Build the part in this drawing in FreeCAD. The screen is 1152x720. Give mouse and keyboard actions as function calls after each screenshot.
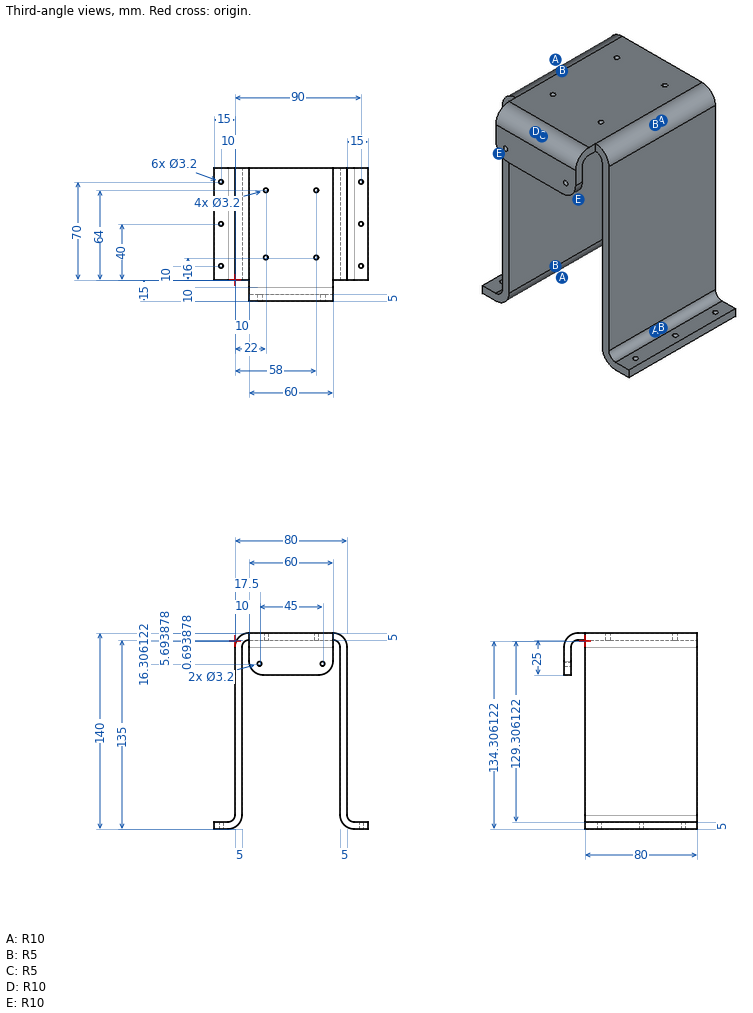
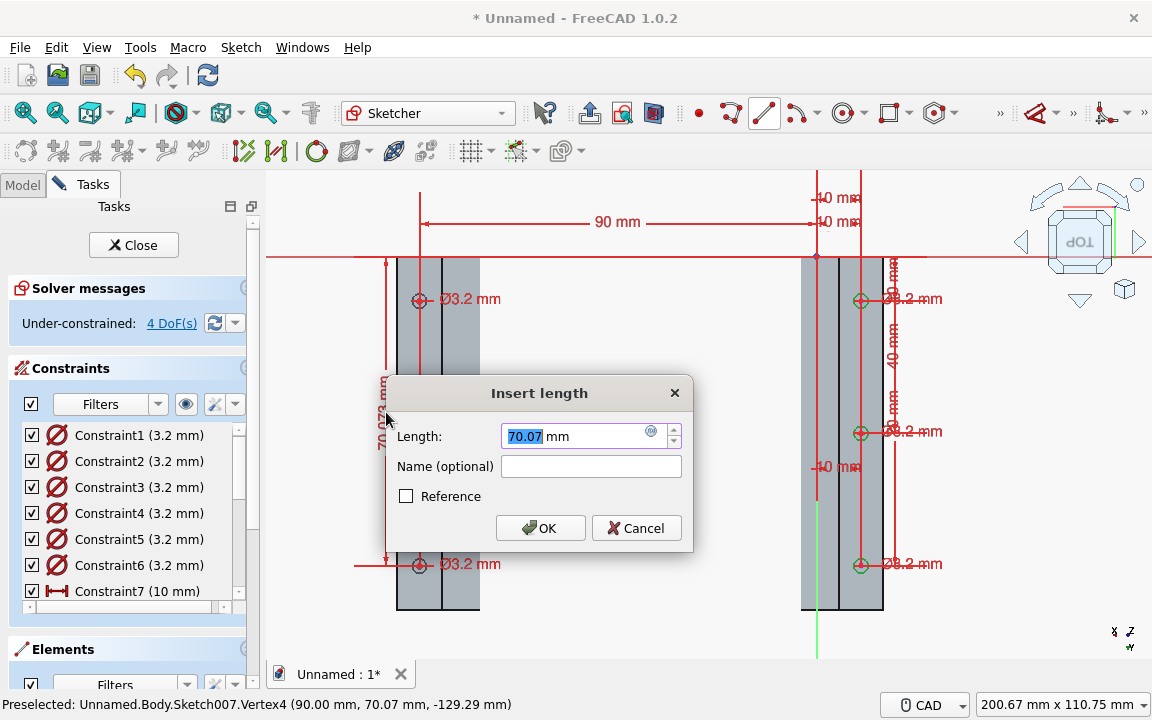
text(70)
key(Return)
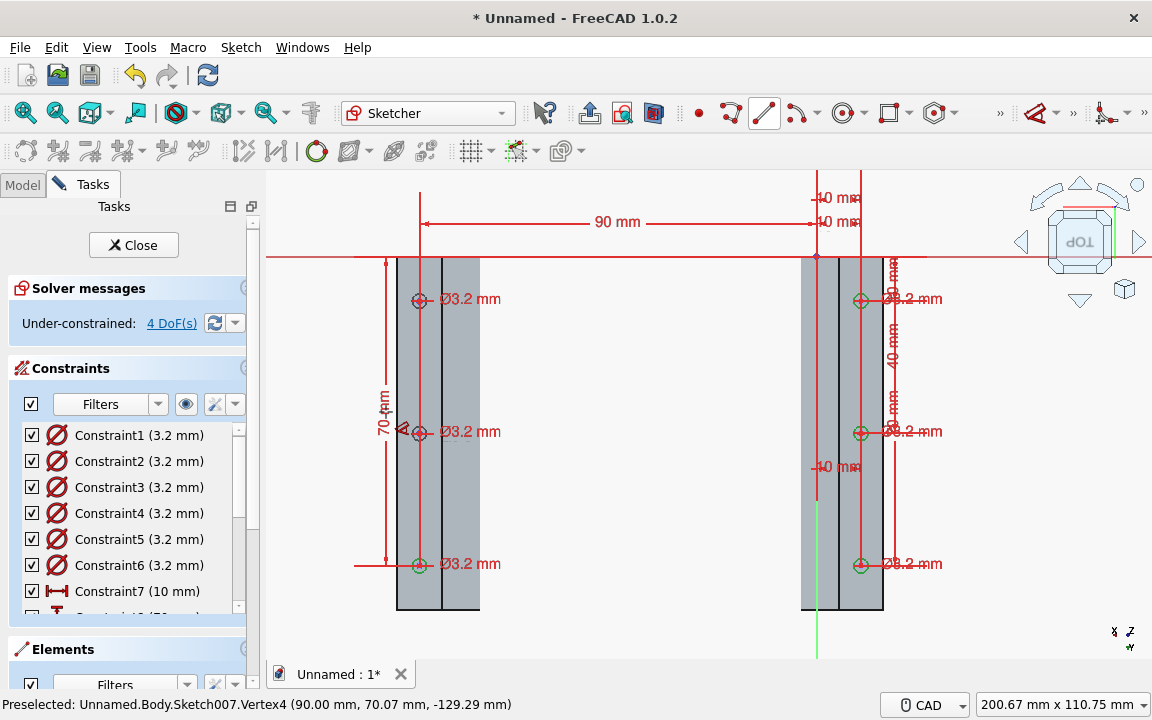
click(420, 434)
click(527, 223)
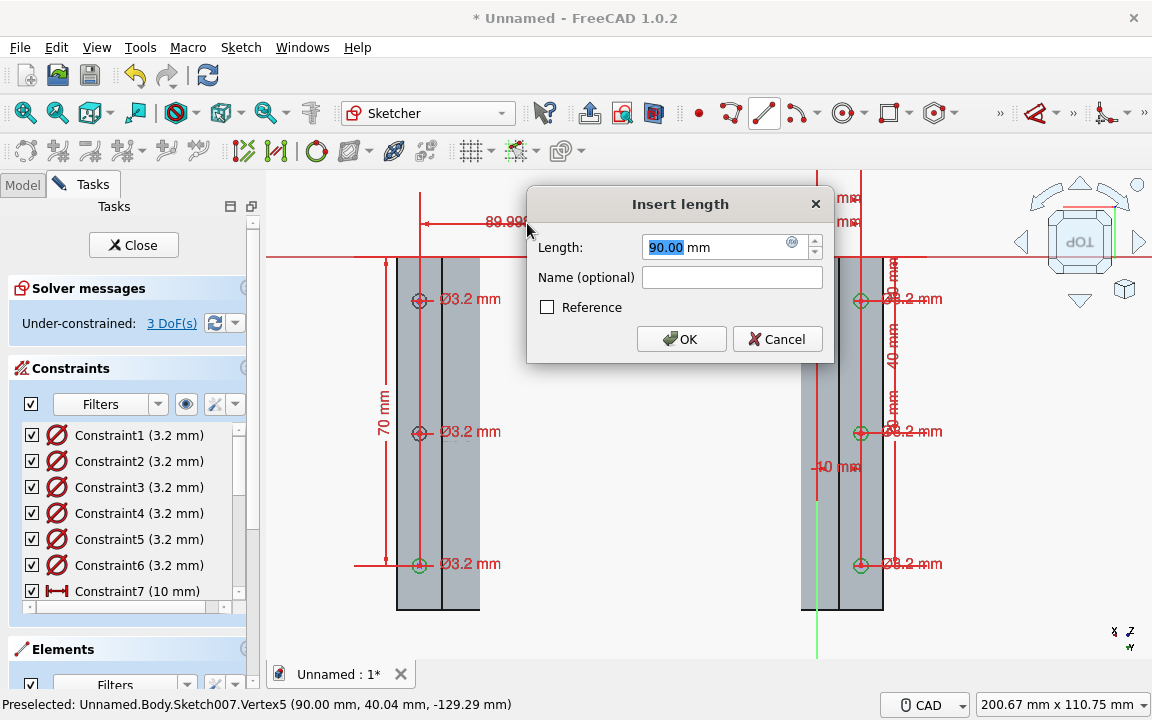
text(90)
key(Return)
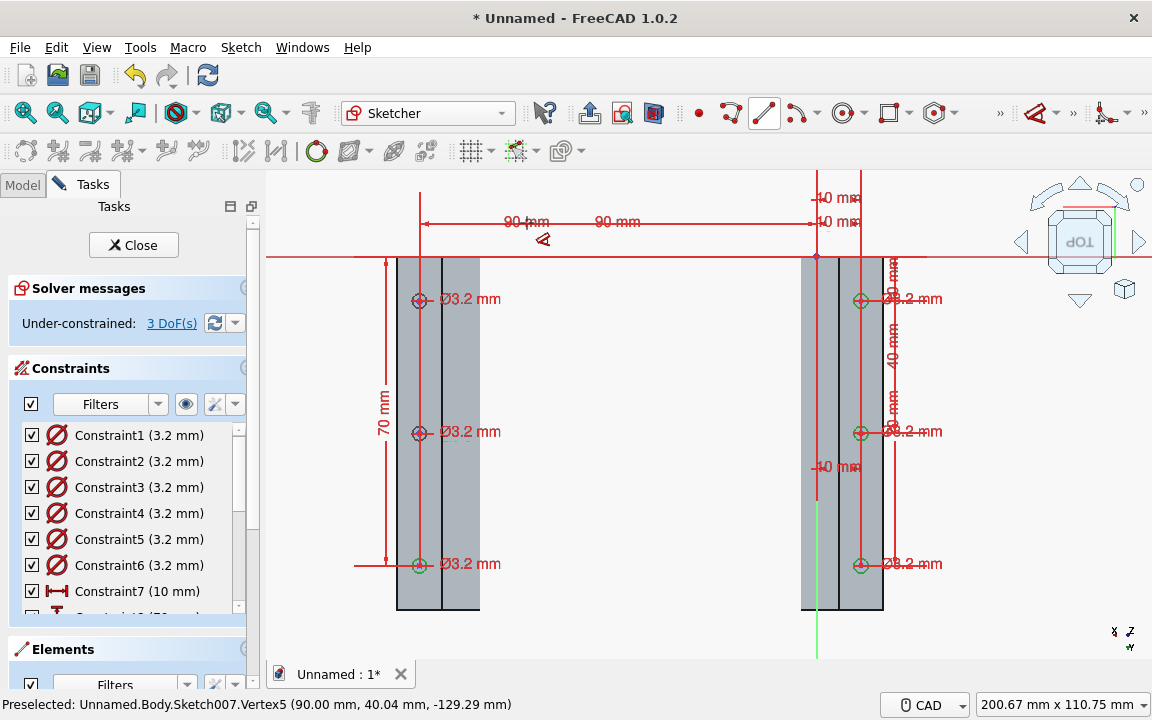
click(420, 434)
click(386, 345)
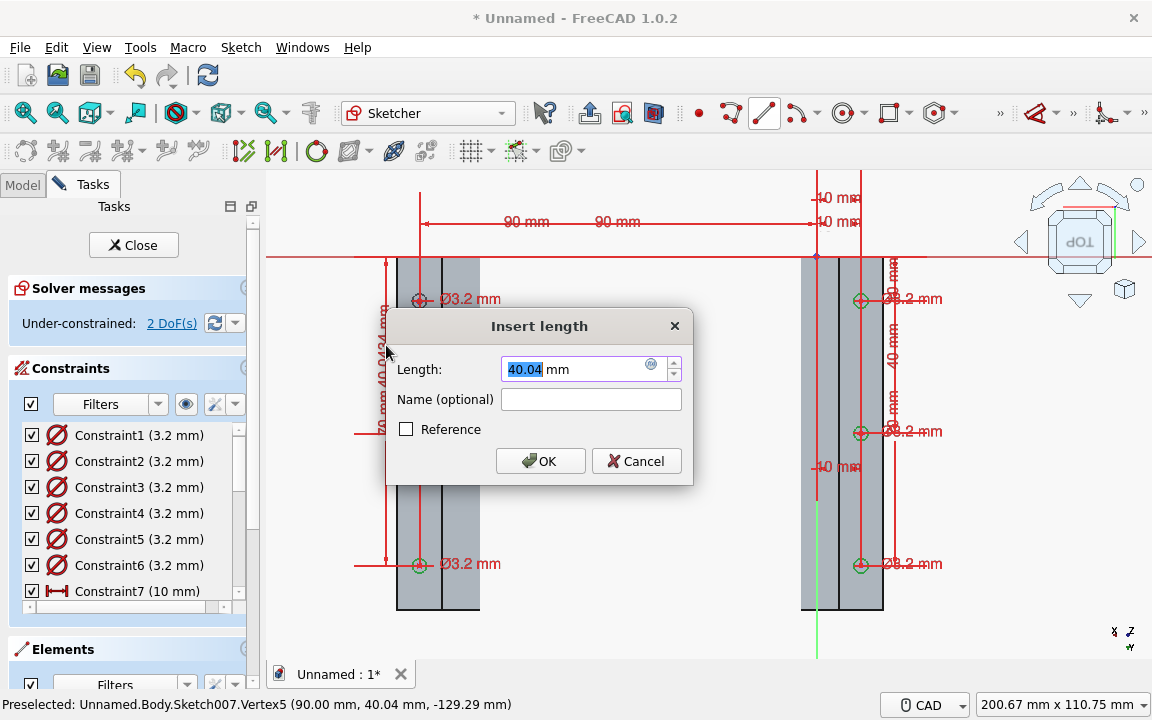
text(40)
key(Return)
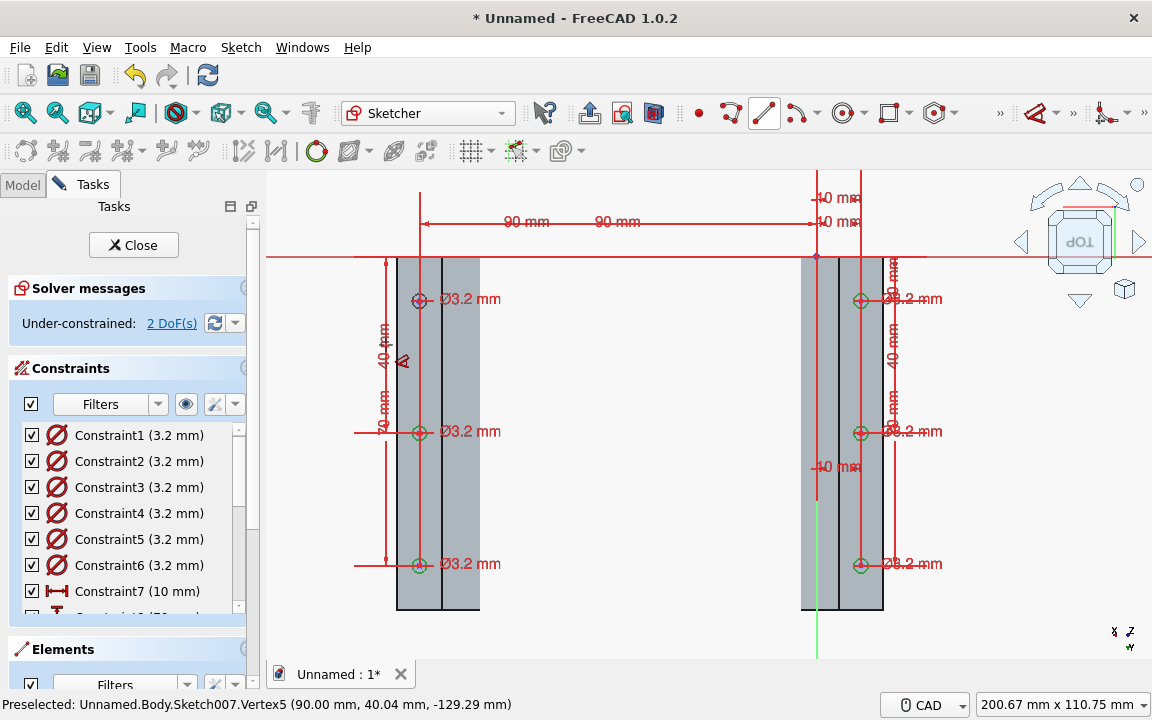
click(420, 301)
click(710, 223)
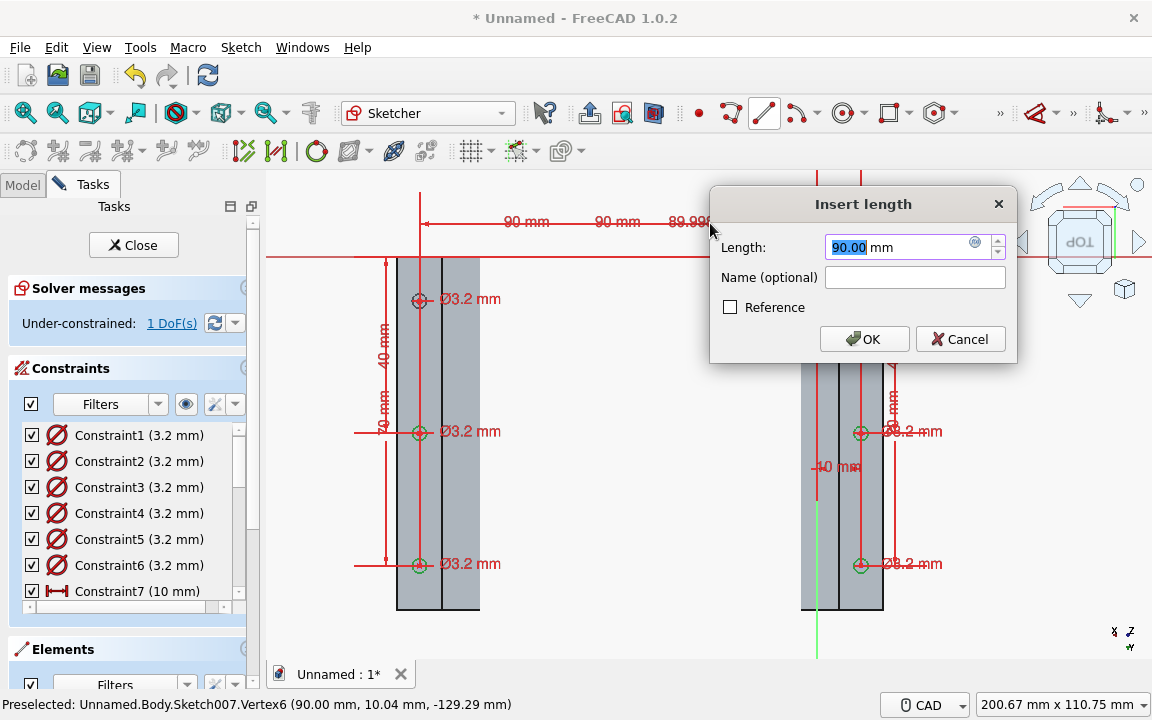
text(90)
key(Return)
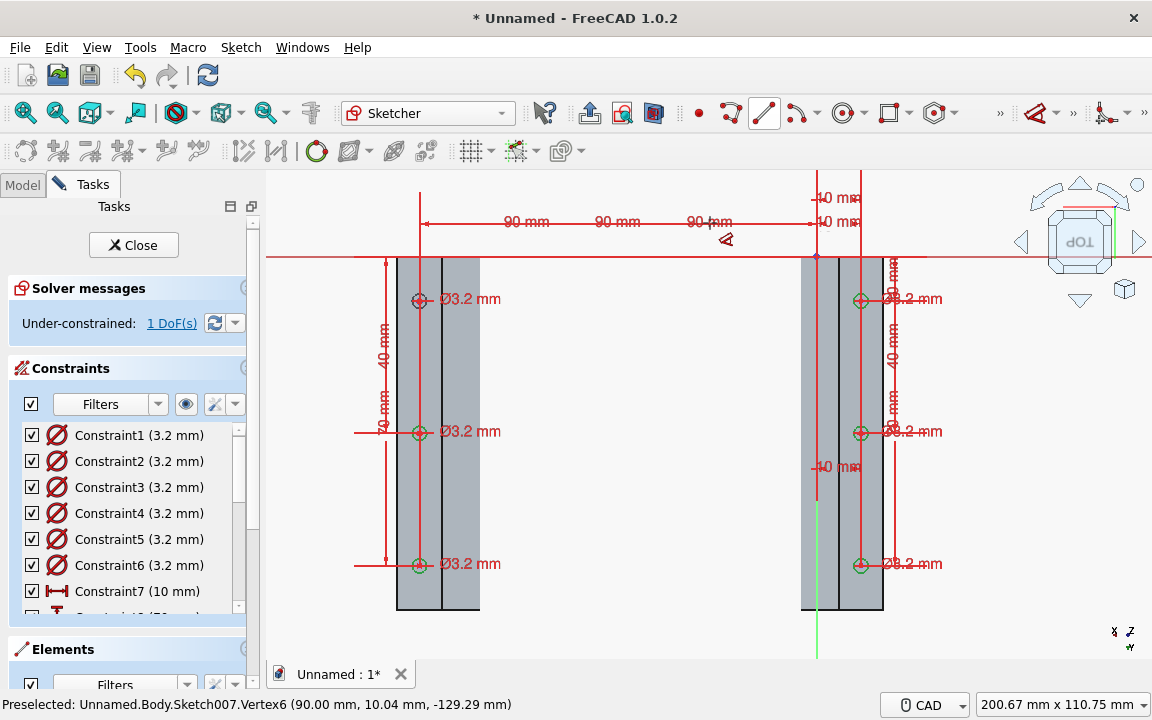
click(420, 301)
click(386, 279)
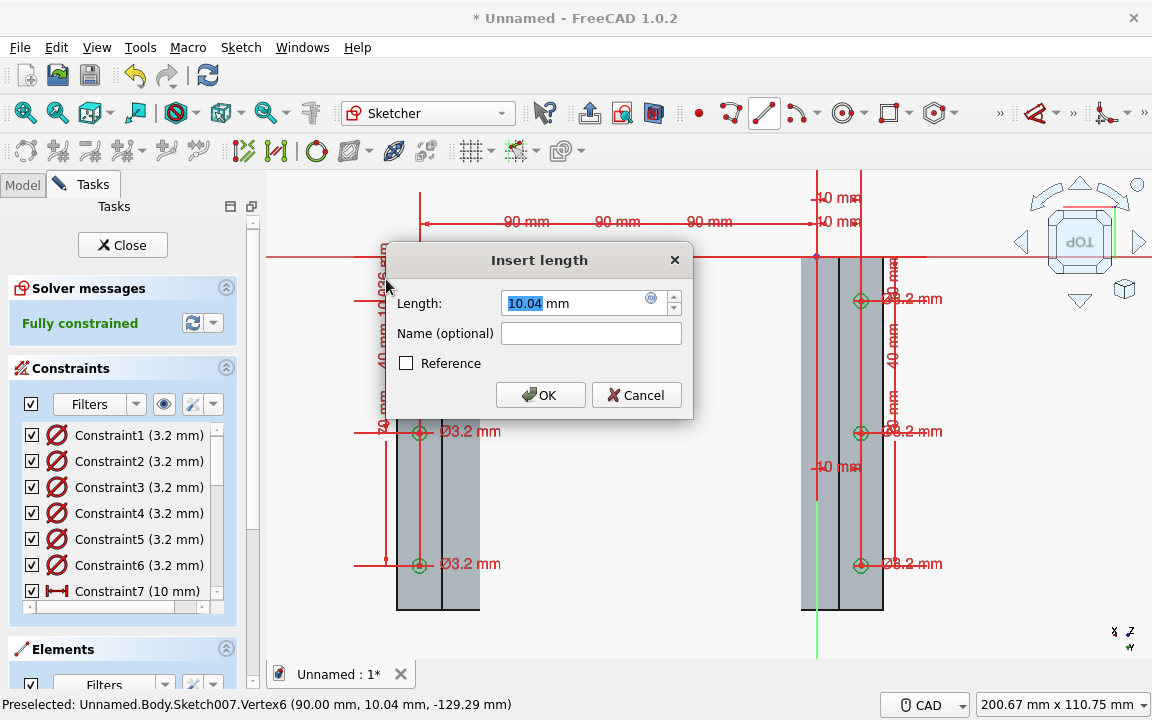
text(10)
key(Return)
key(Escape)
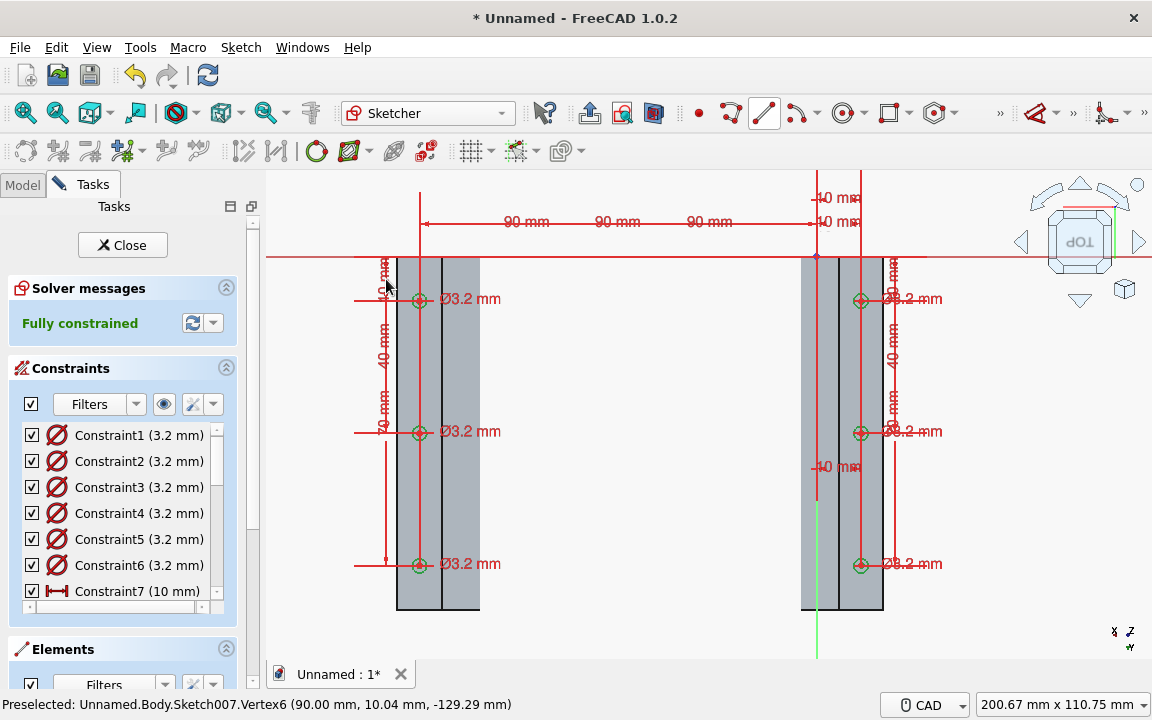
click(123, 245)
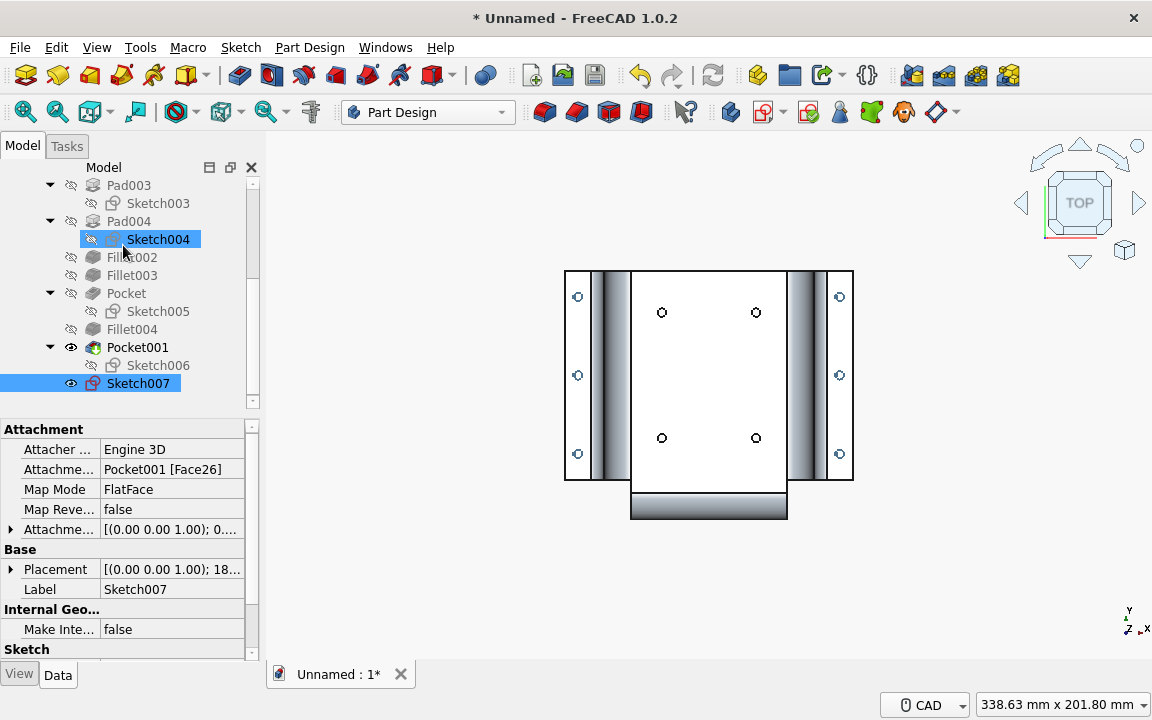
click(240, 76)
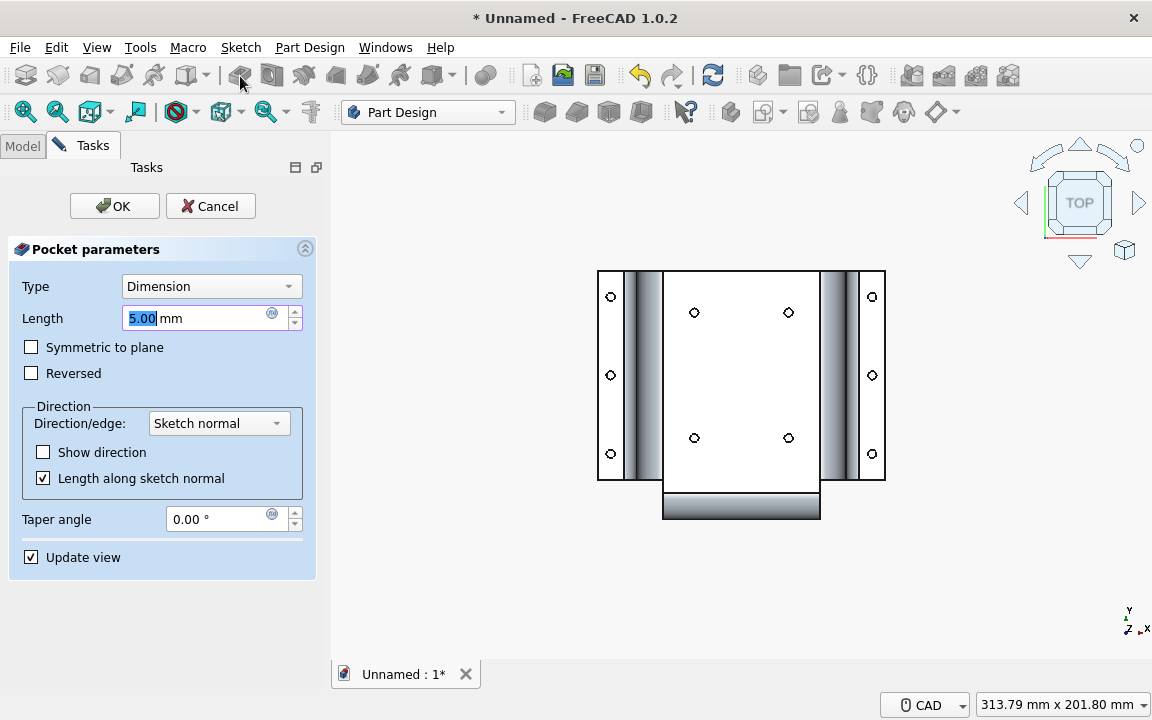
click(212, 286)